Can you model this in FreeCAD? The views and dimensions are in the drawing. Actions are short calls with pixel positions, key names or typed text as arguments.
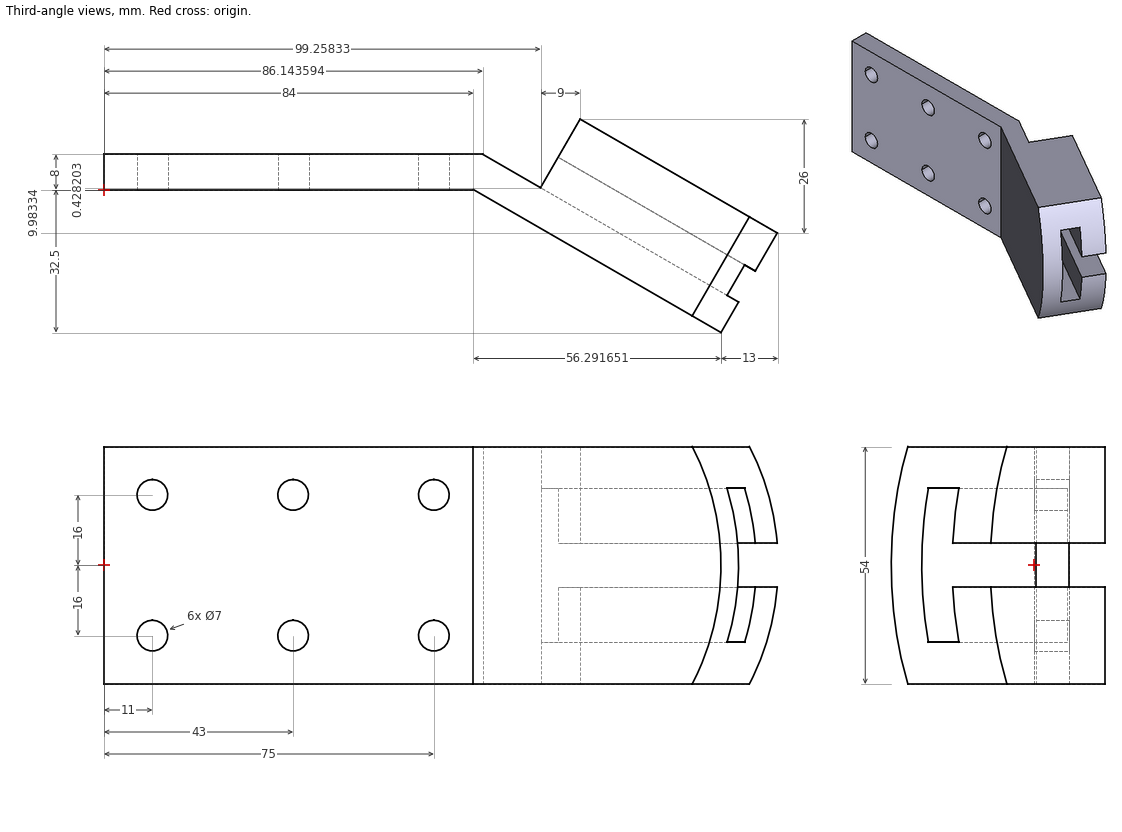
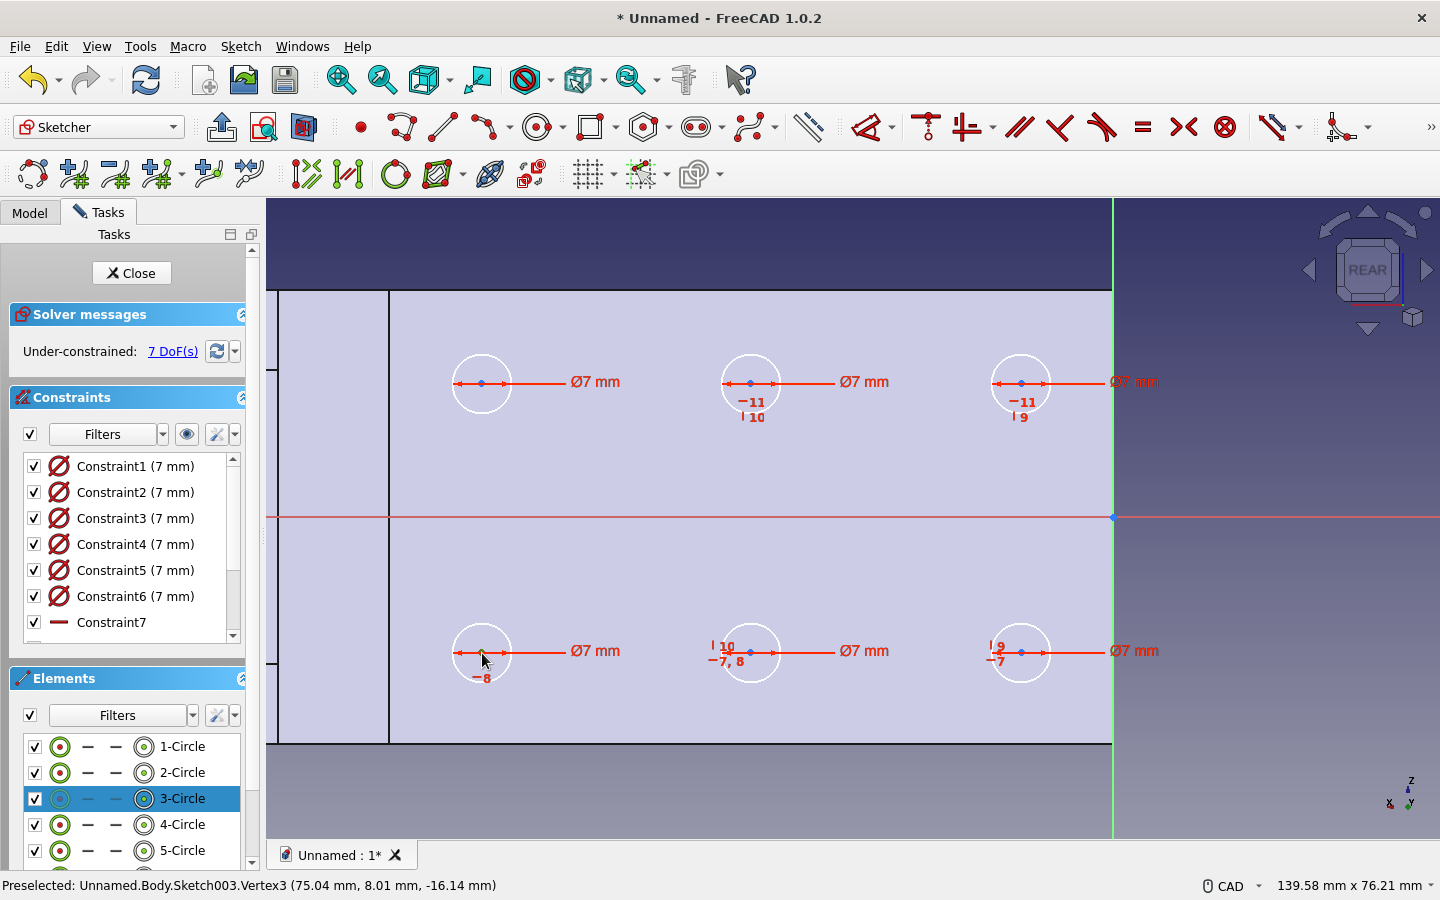
click(482, 384)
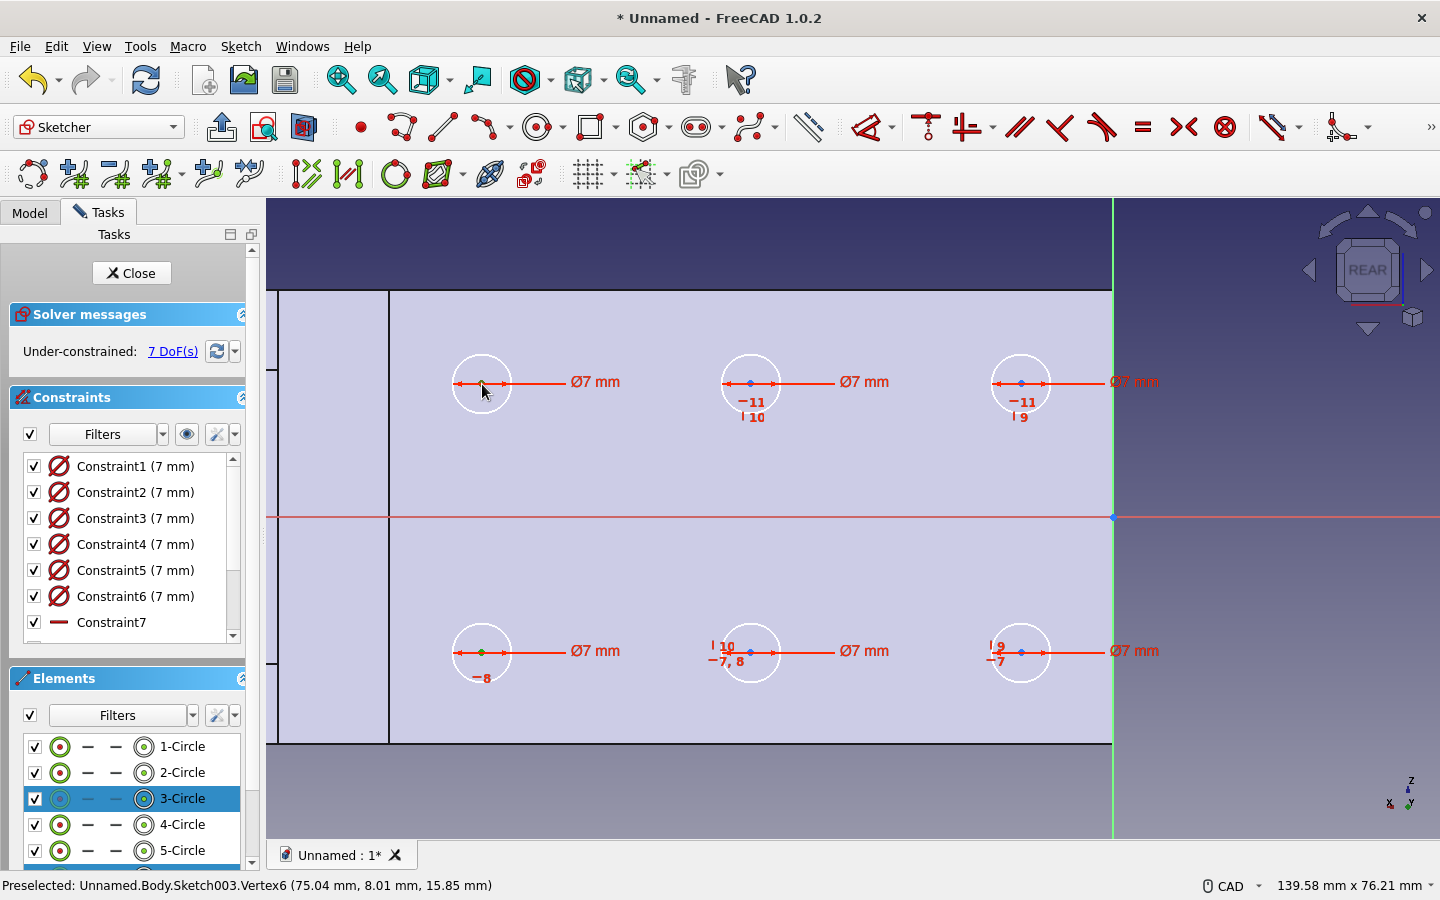
key(v)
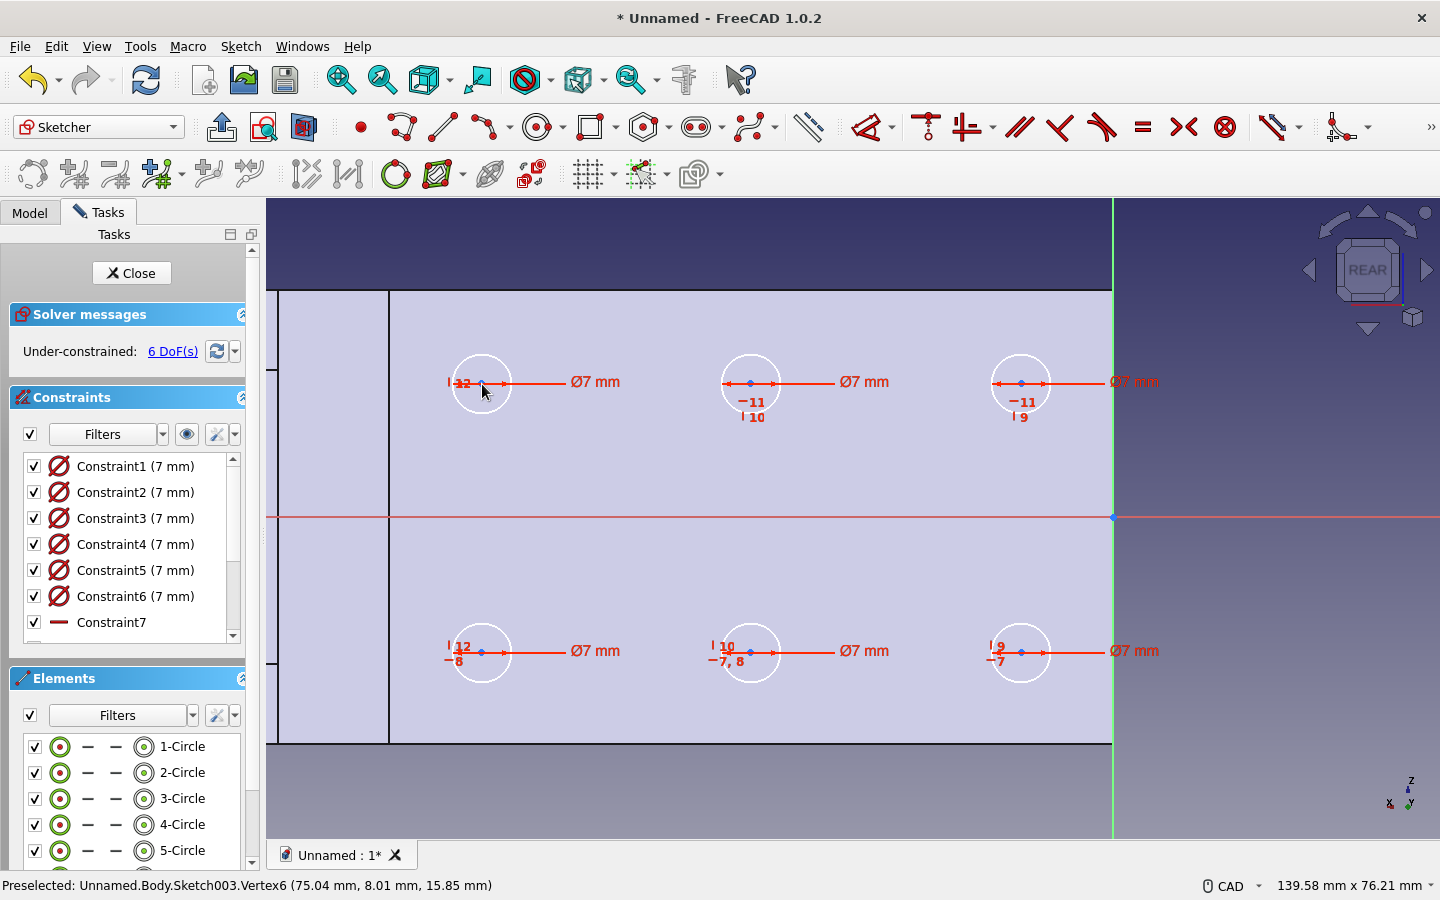
click(751, 384)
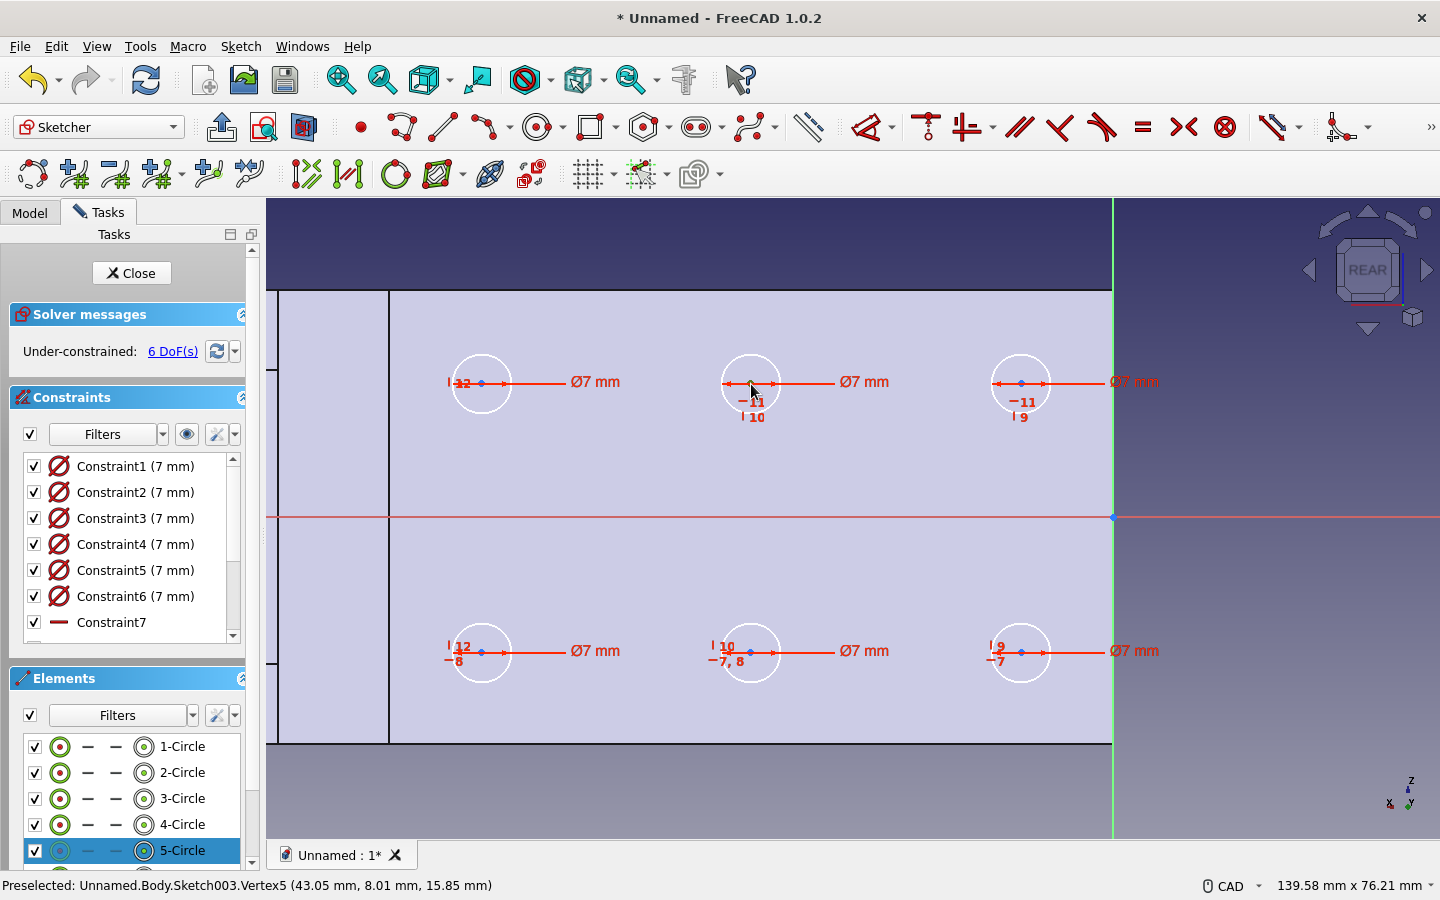
click(482, 384)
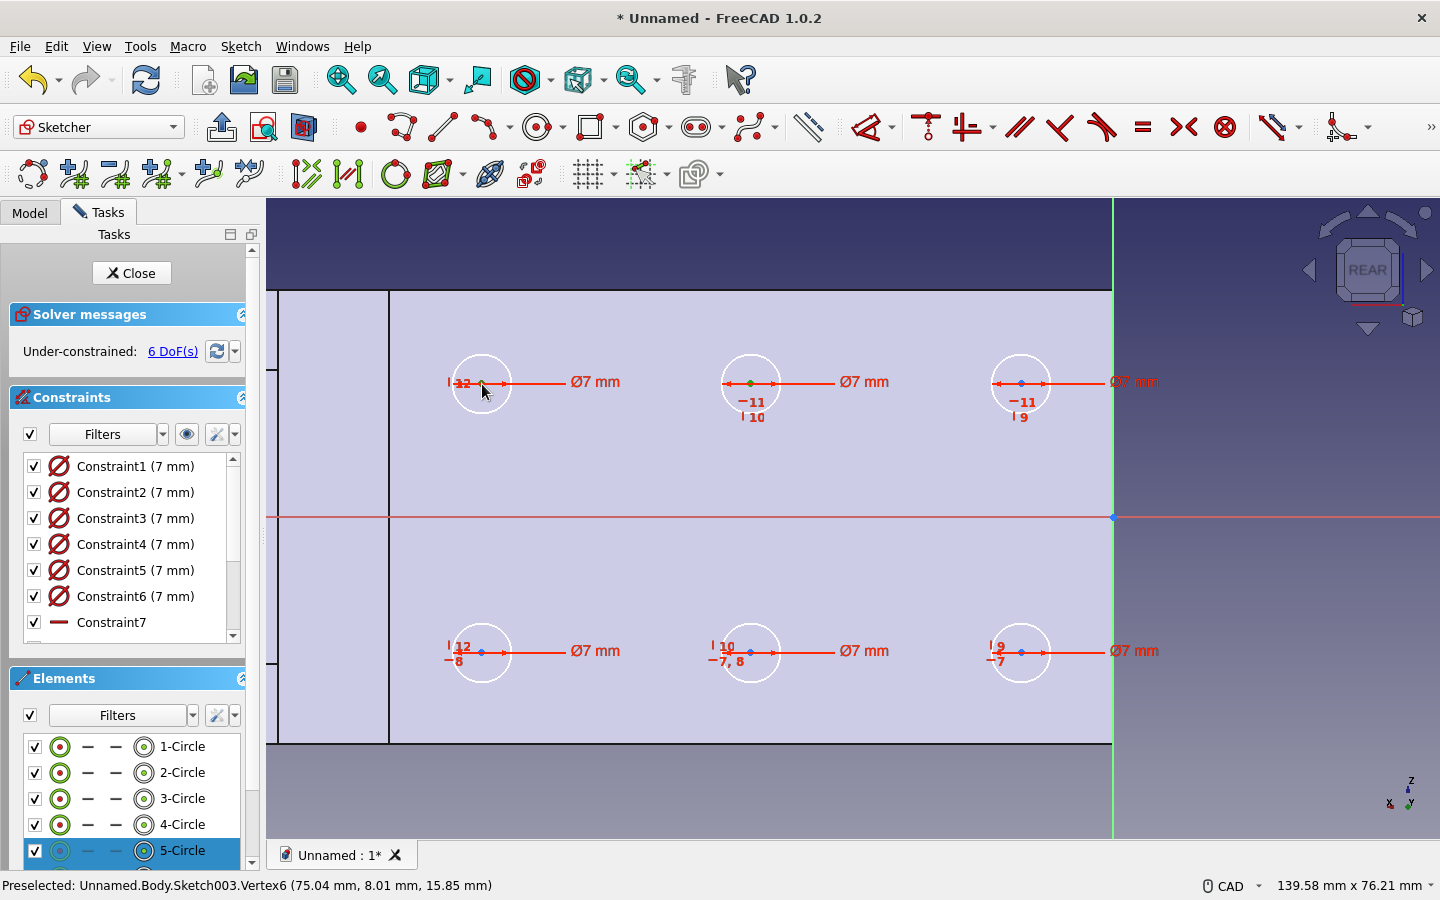
key(h)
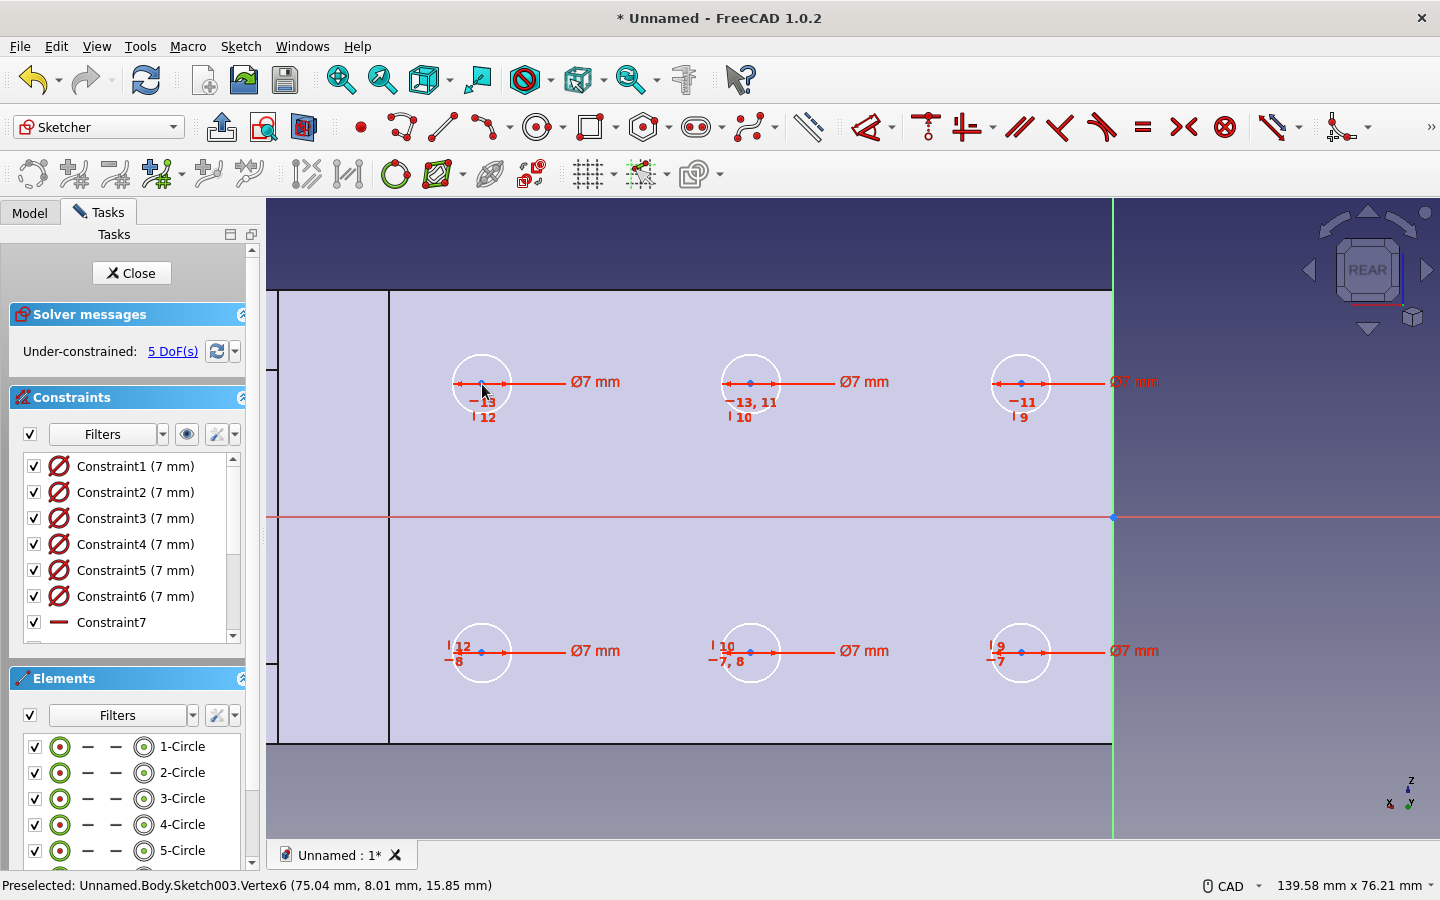
key(d)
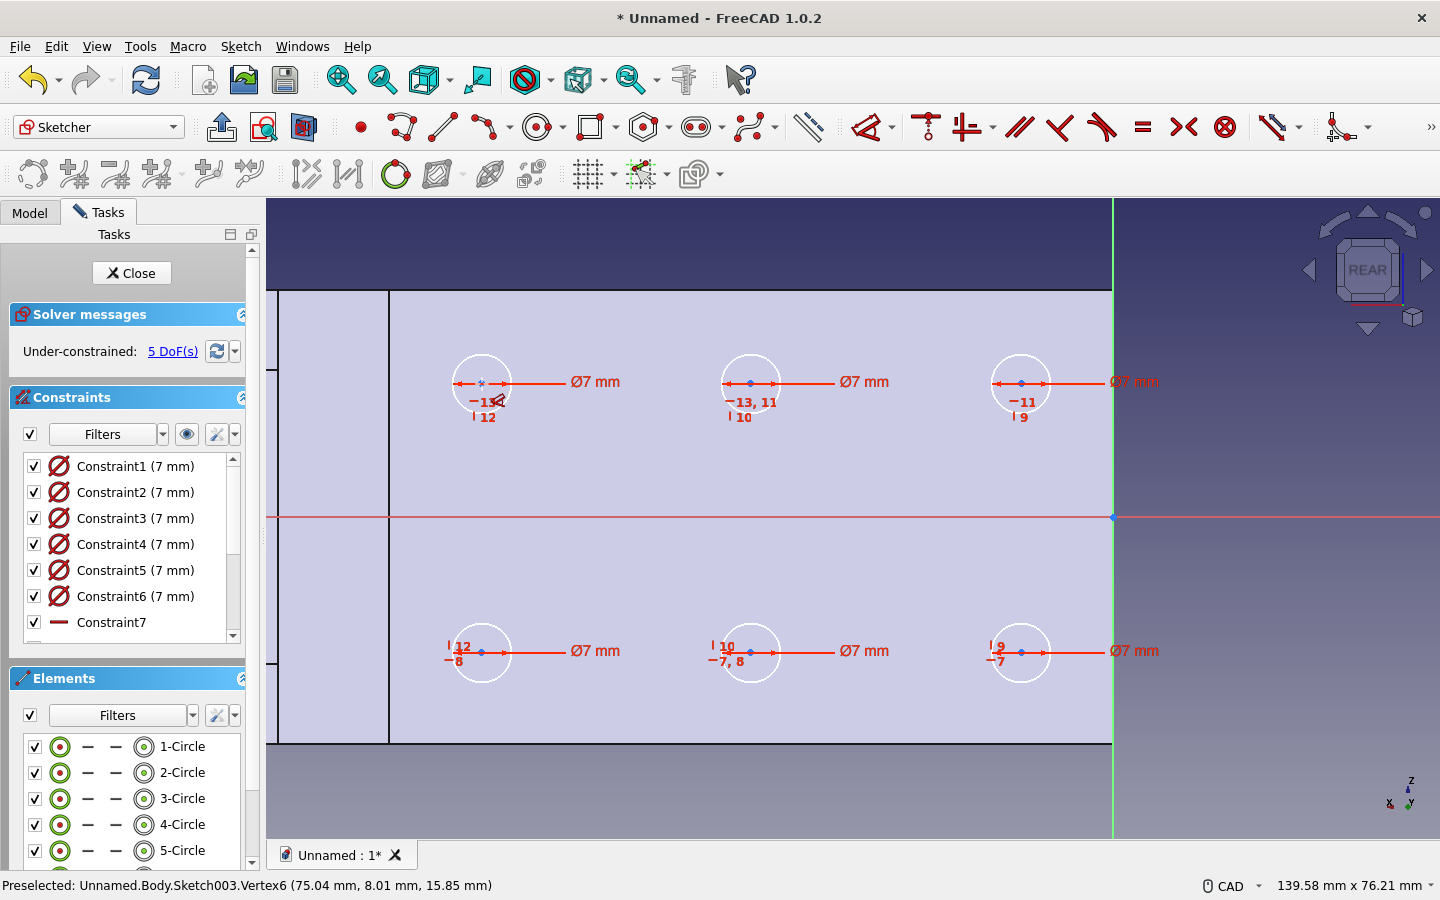
click(1021, 653)
click(1067, 687)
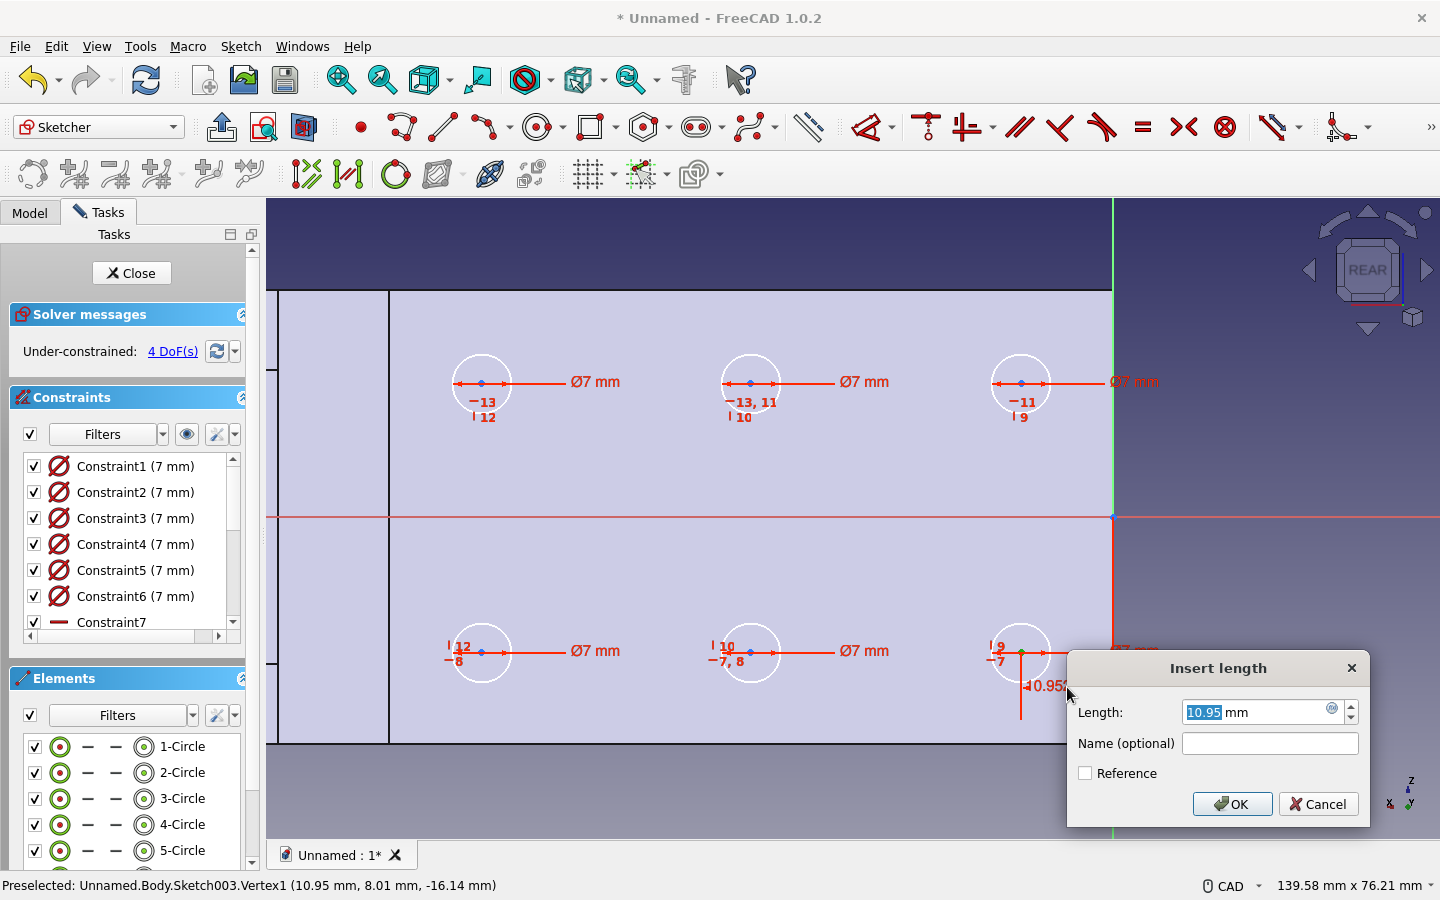
text(11)
key(Return)